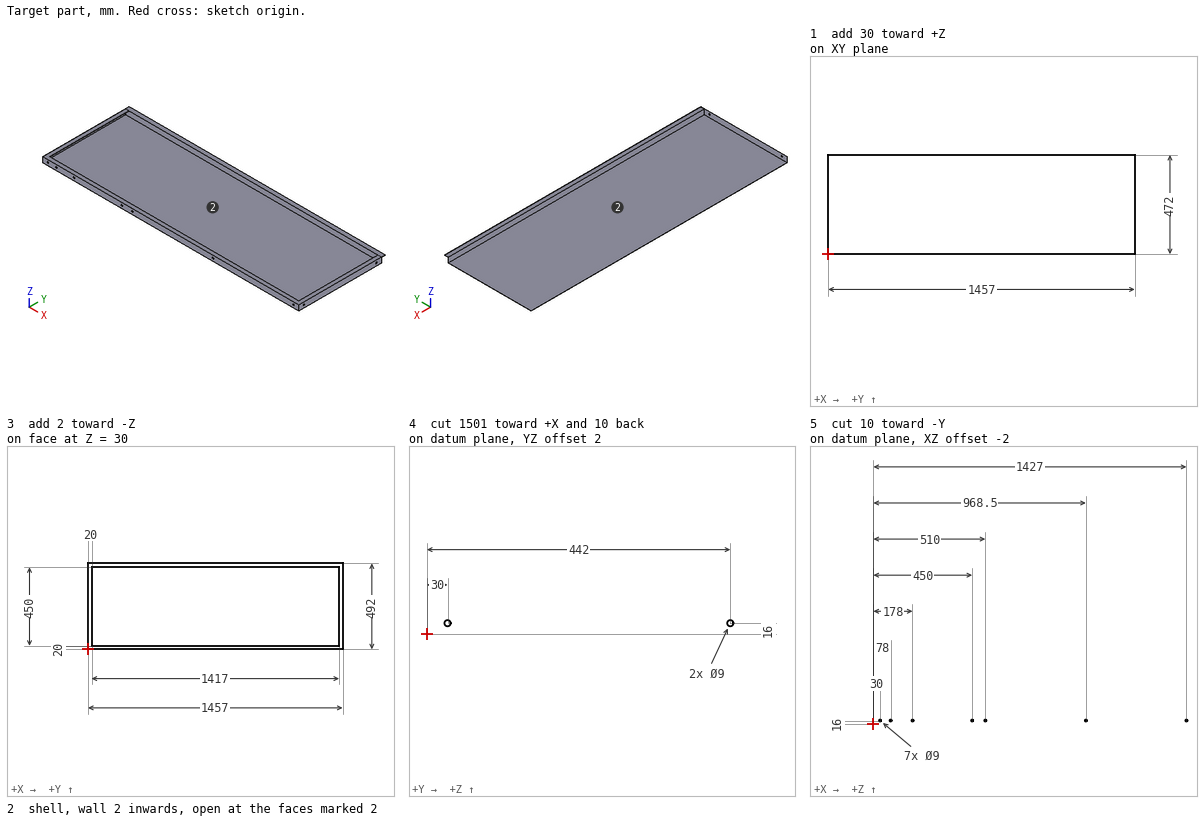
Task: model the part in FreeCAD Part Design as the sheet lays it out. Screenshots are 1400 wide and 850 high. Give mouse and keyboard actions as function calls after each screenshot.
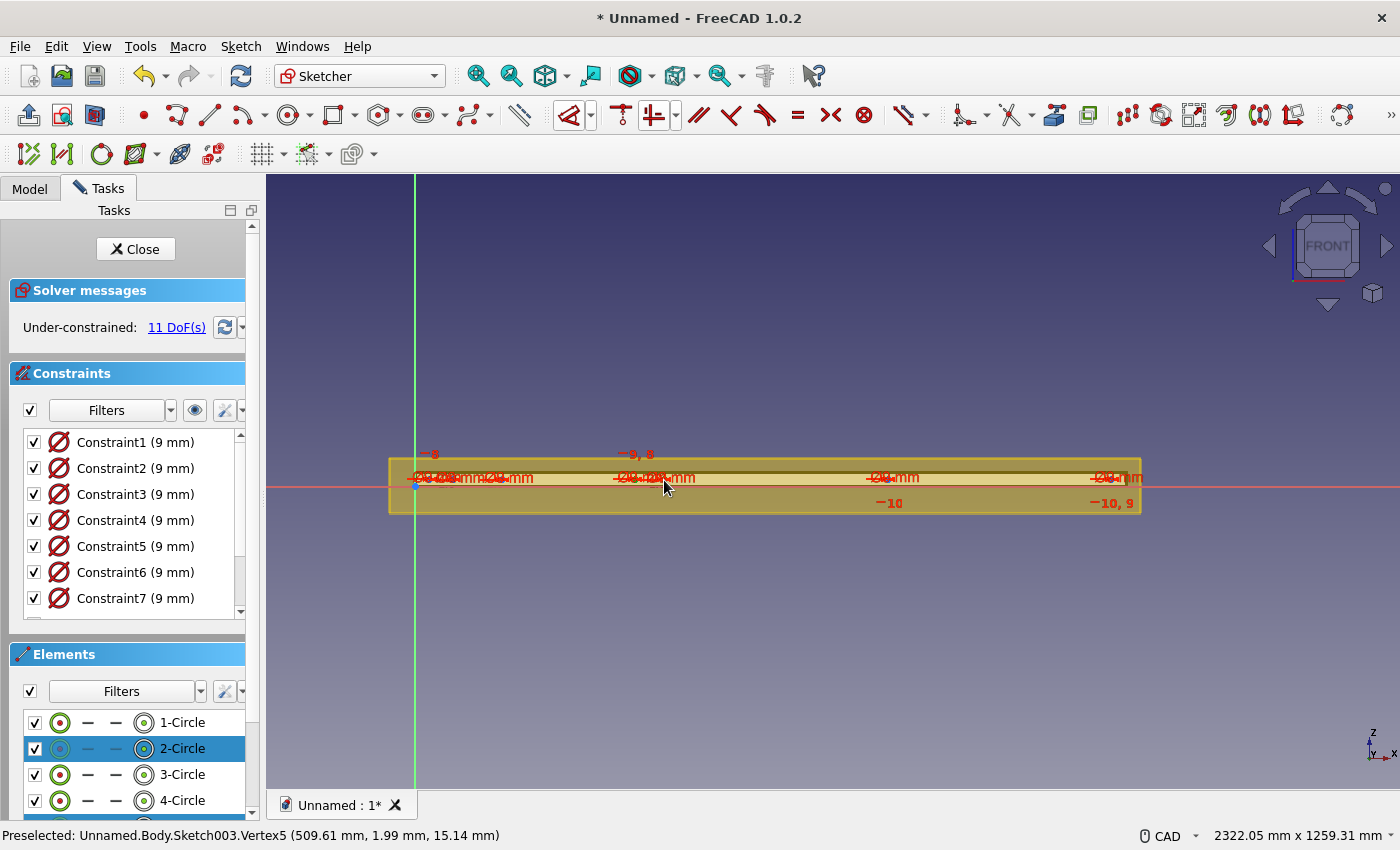
key(h)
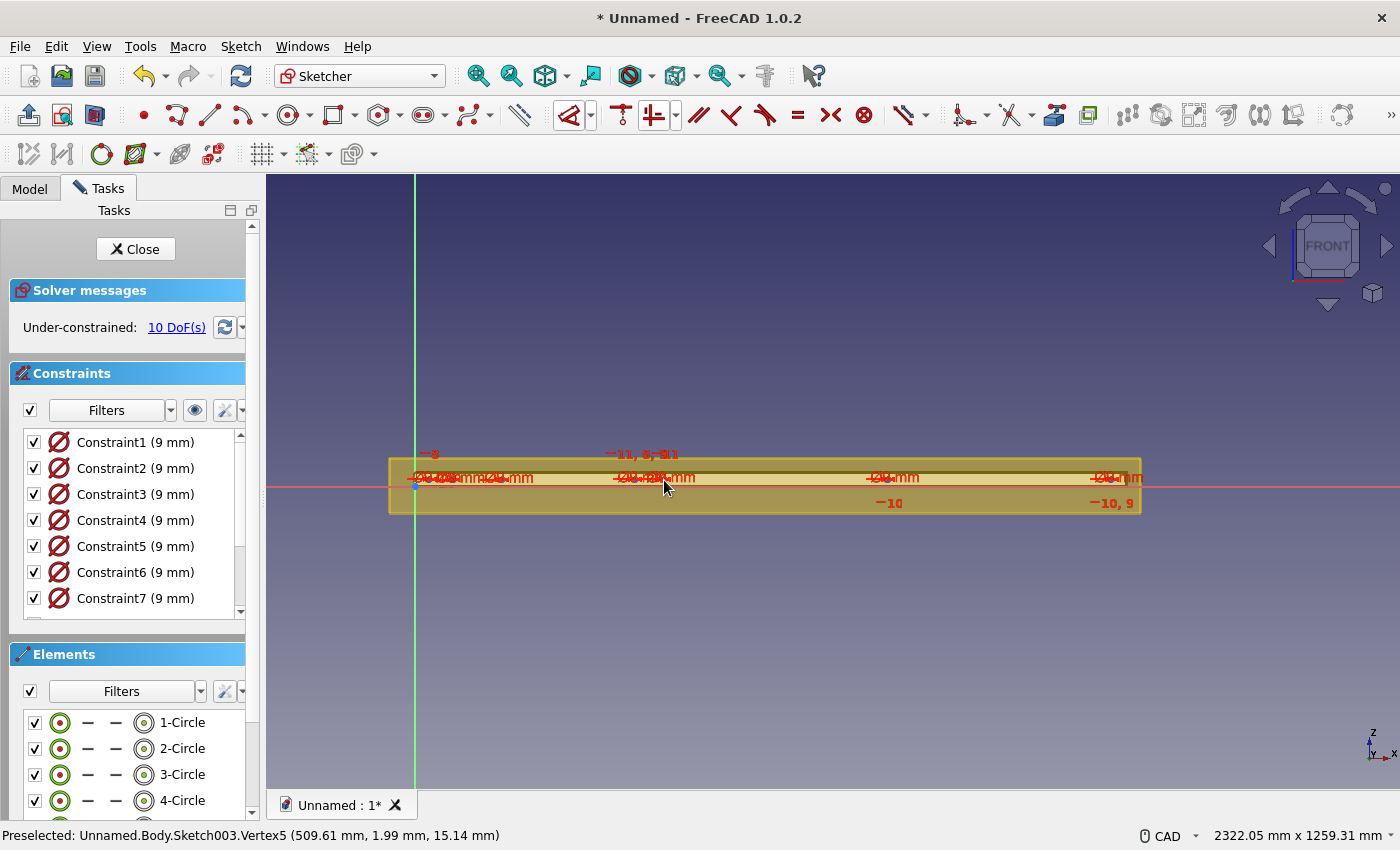
click(430, 479)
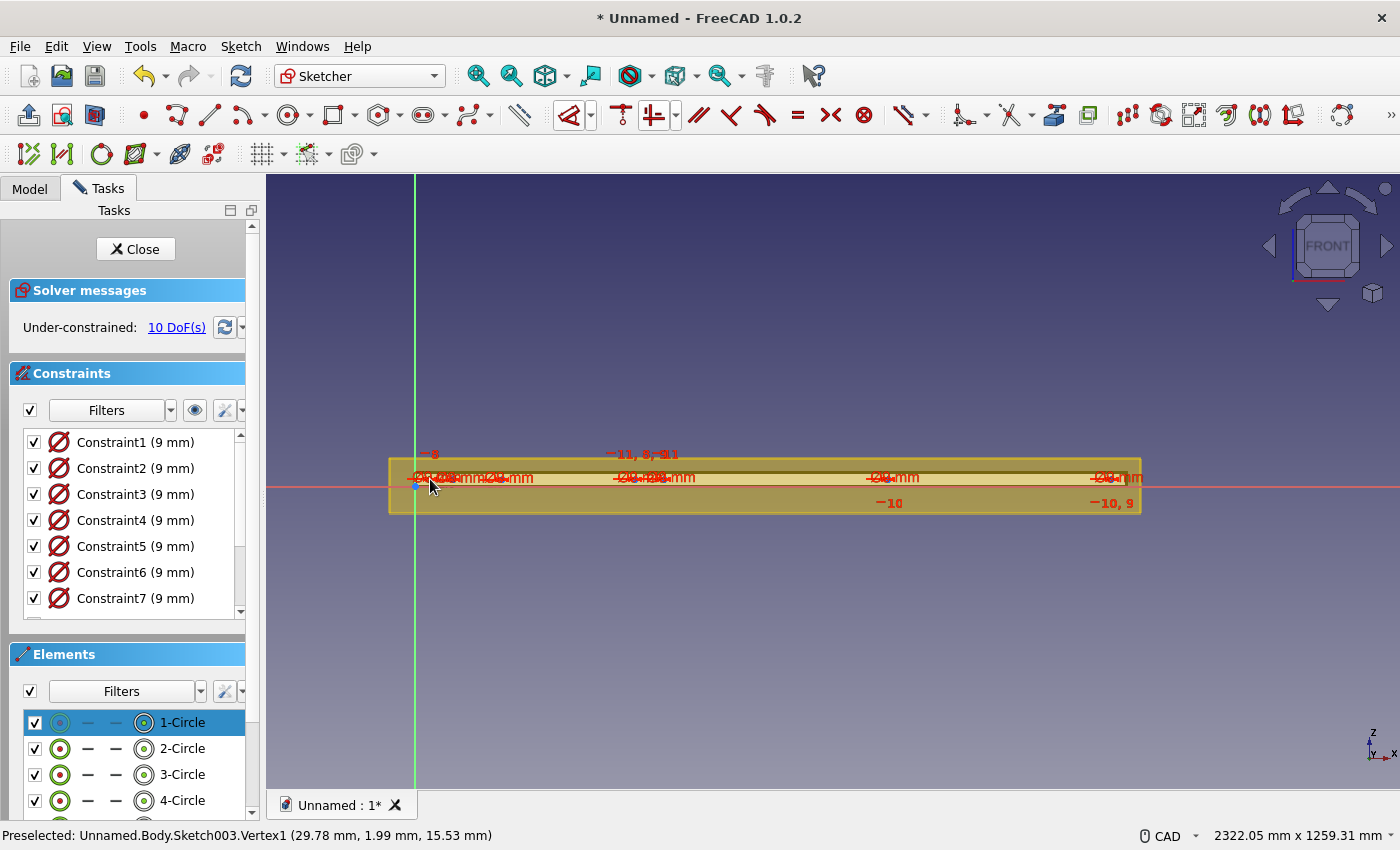
click(453, 480)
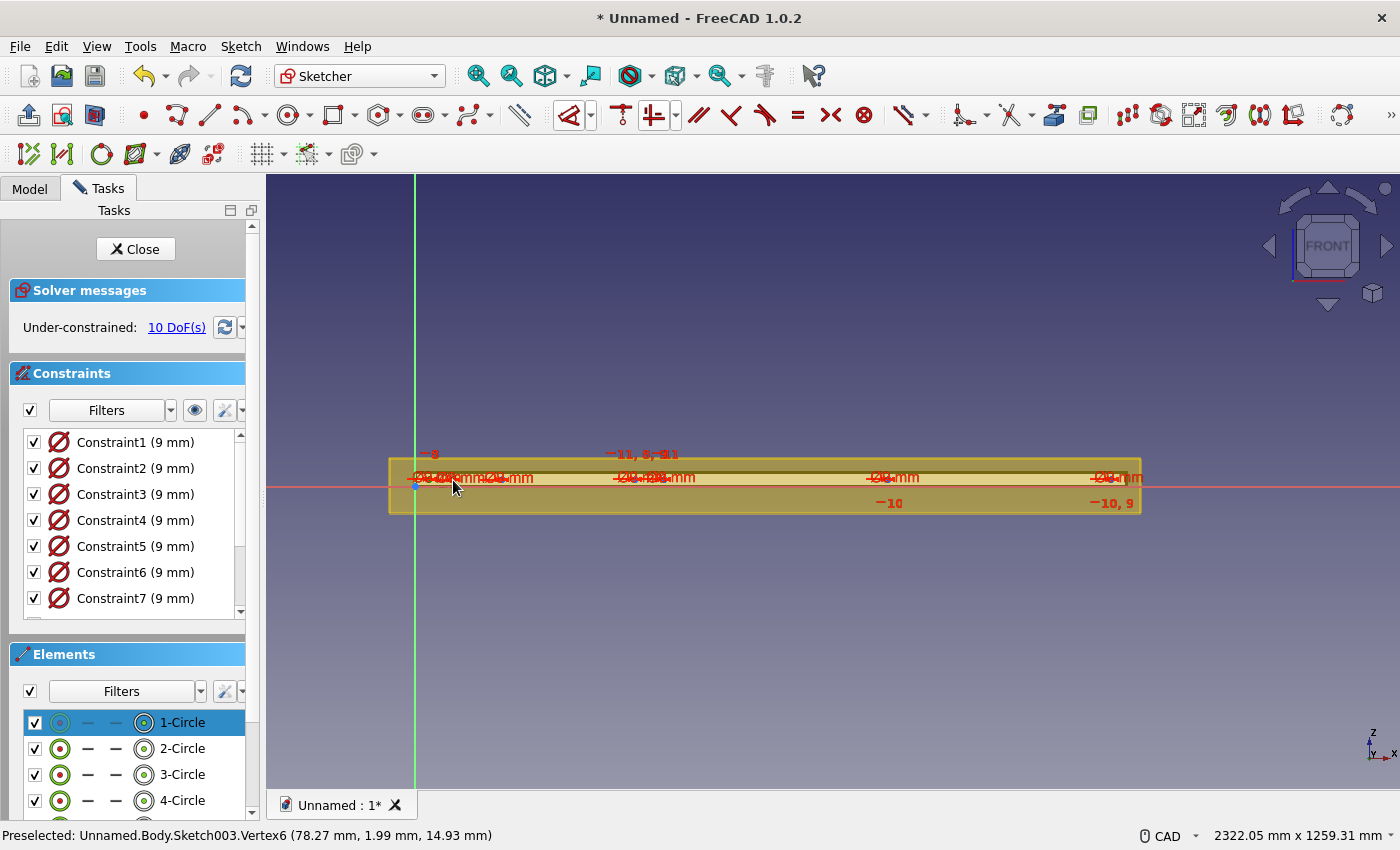
click(676, 116)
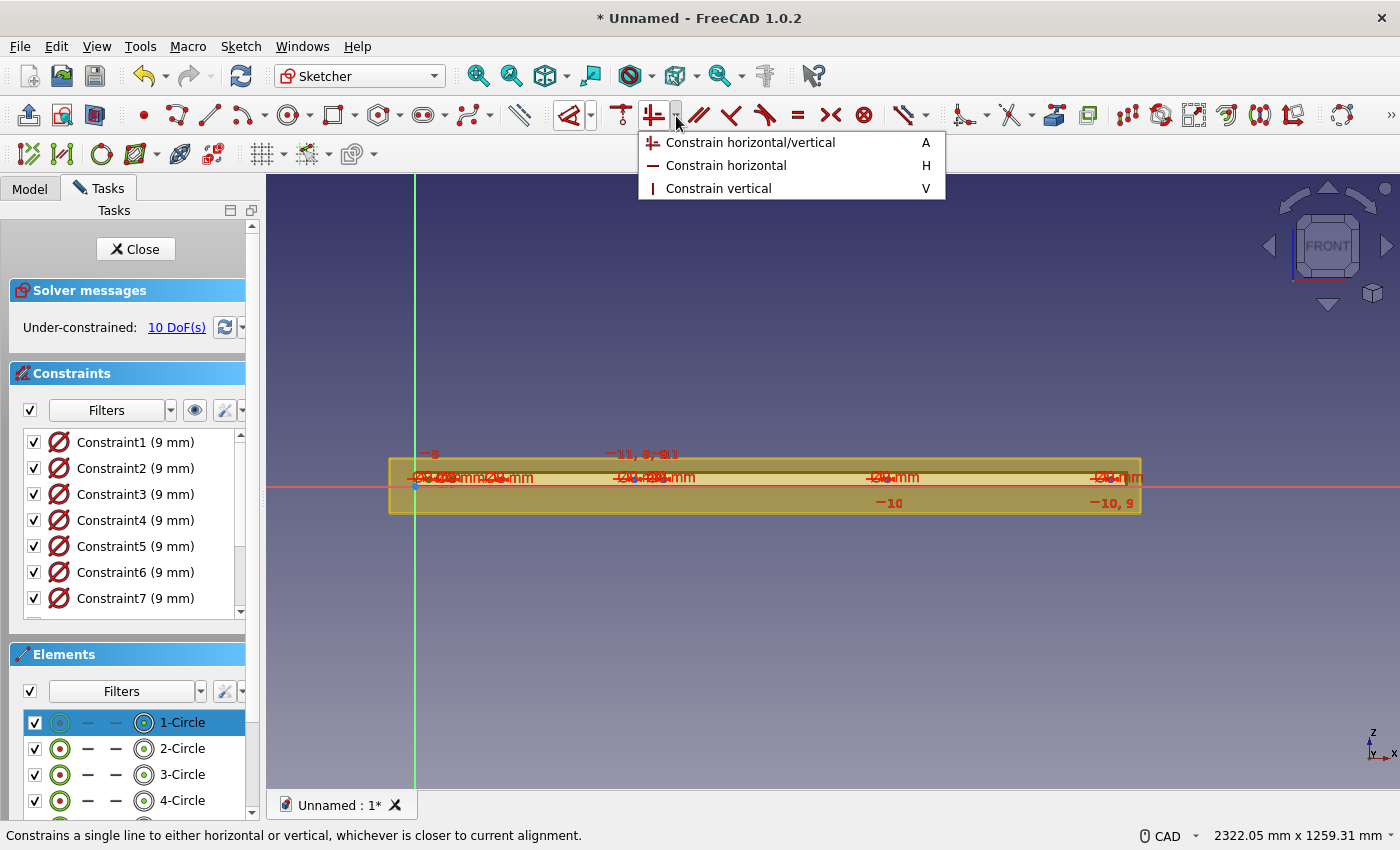
click(792, 166)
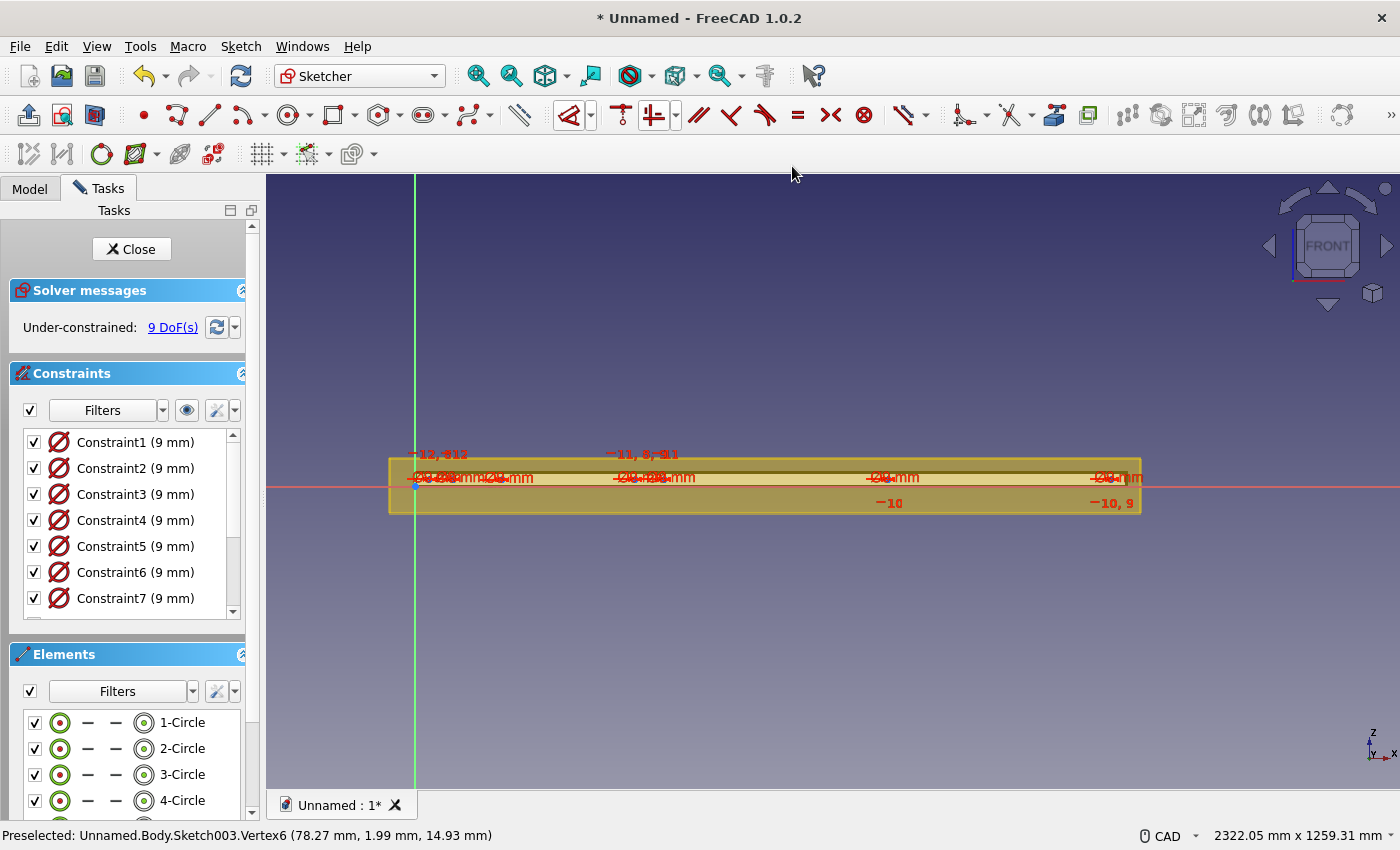
click(453, 479)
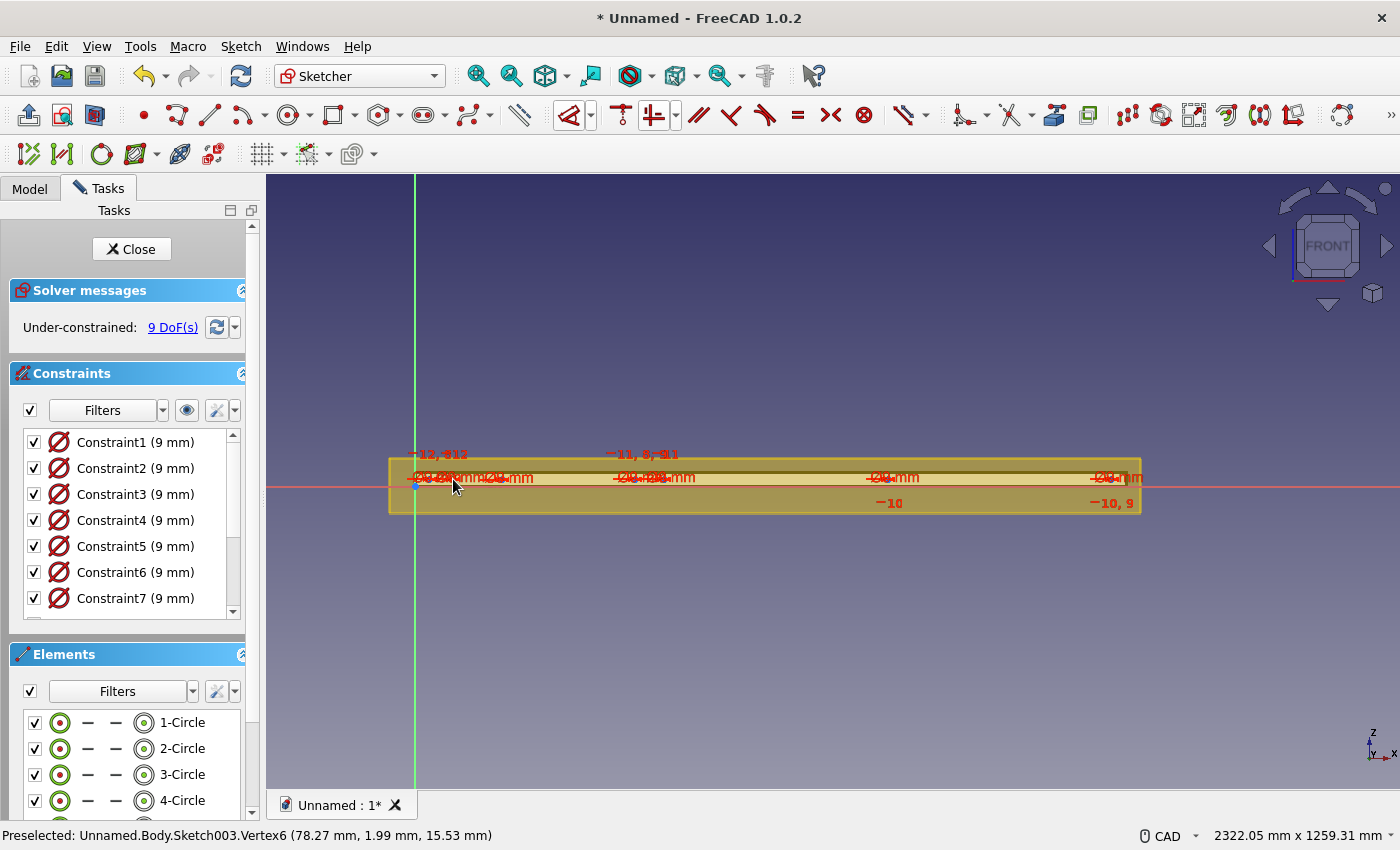
click(502, 480)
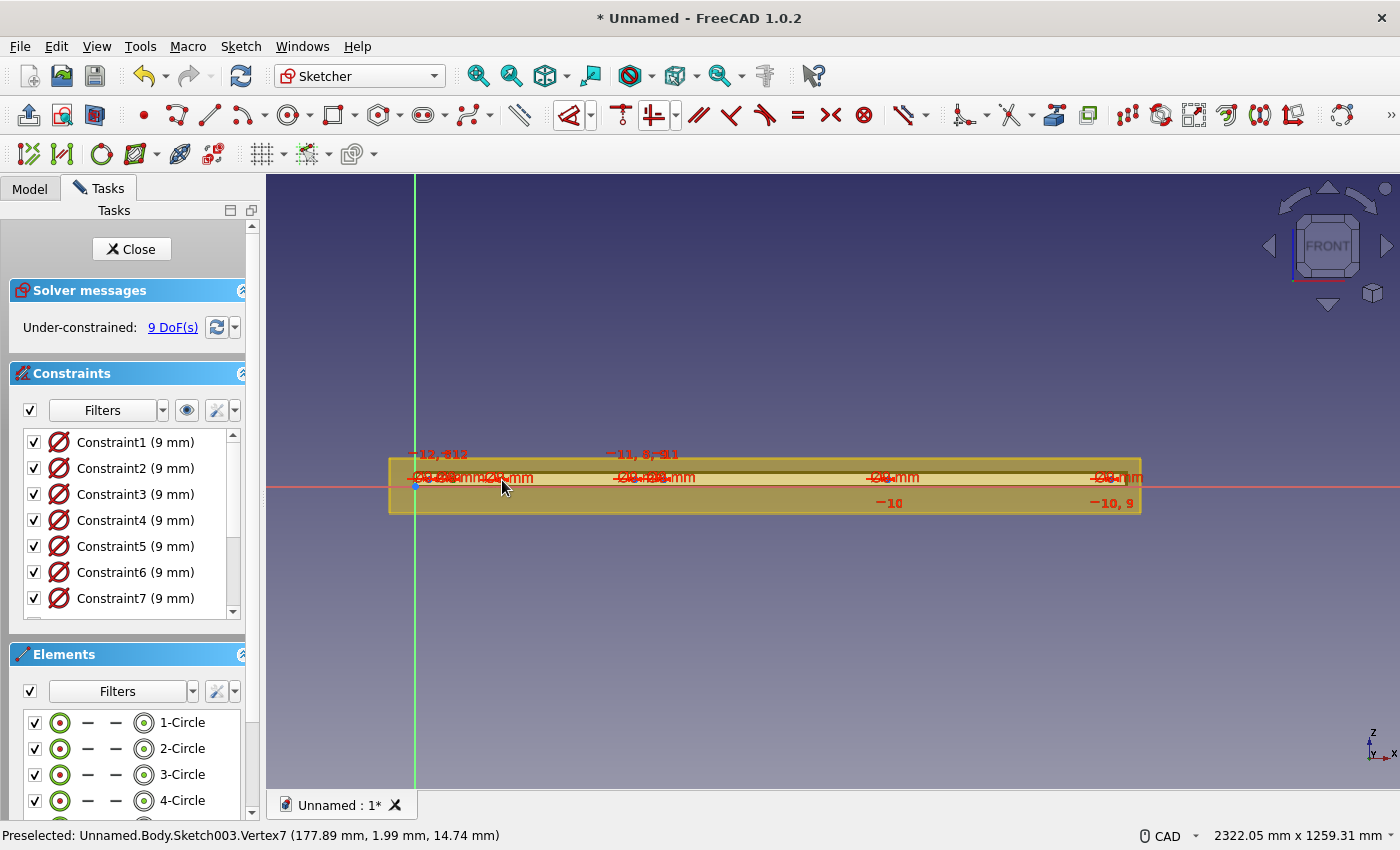
key(h)